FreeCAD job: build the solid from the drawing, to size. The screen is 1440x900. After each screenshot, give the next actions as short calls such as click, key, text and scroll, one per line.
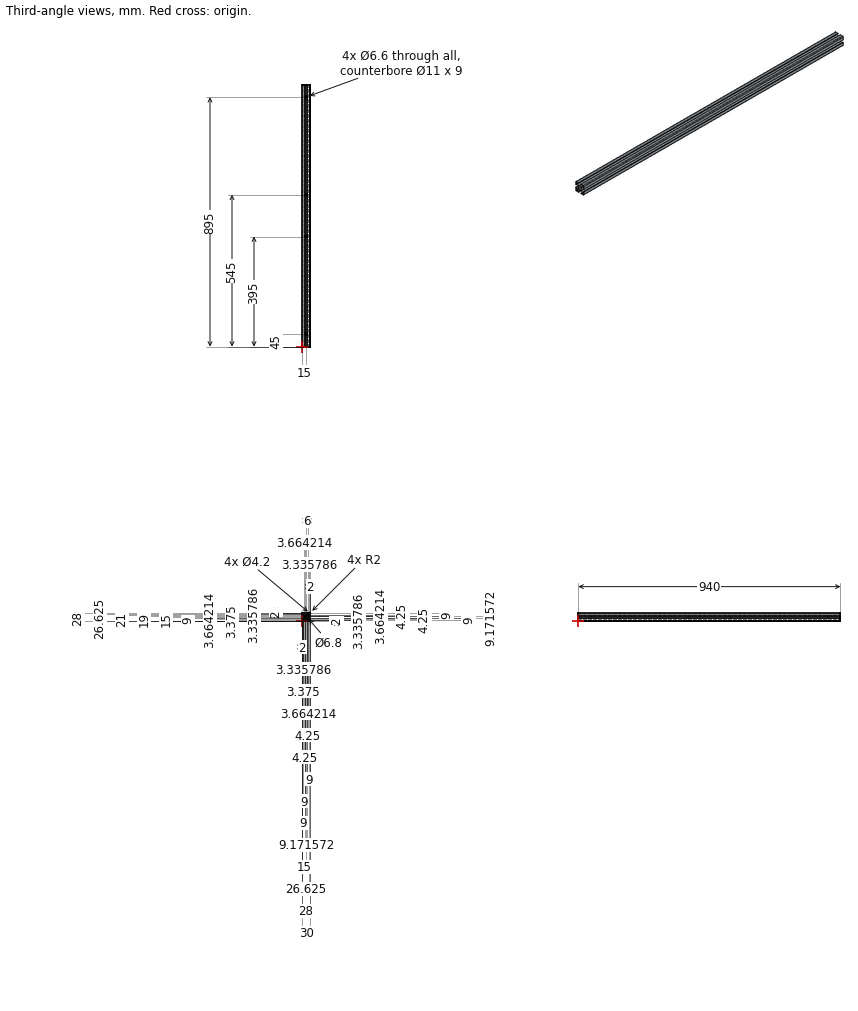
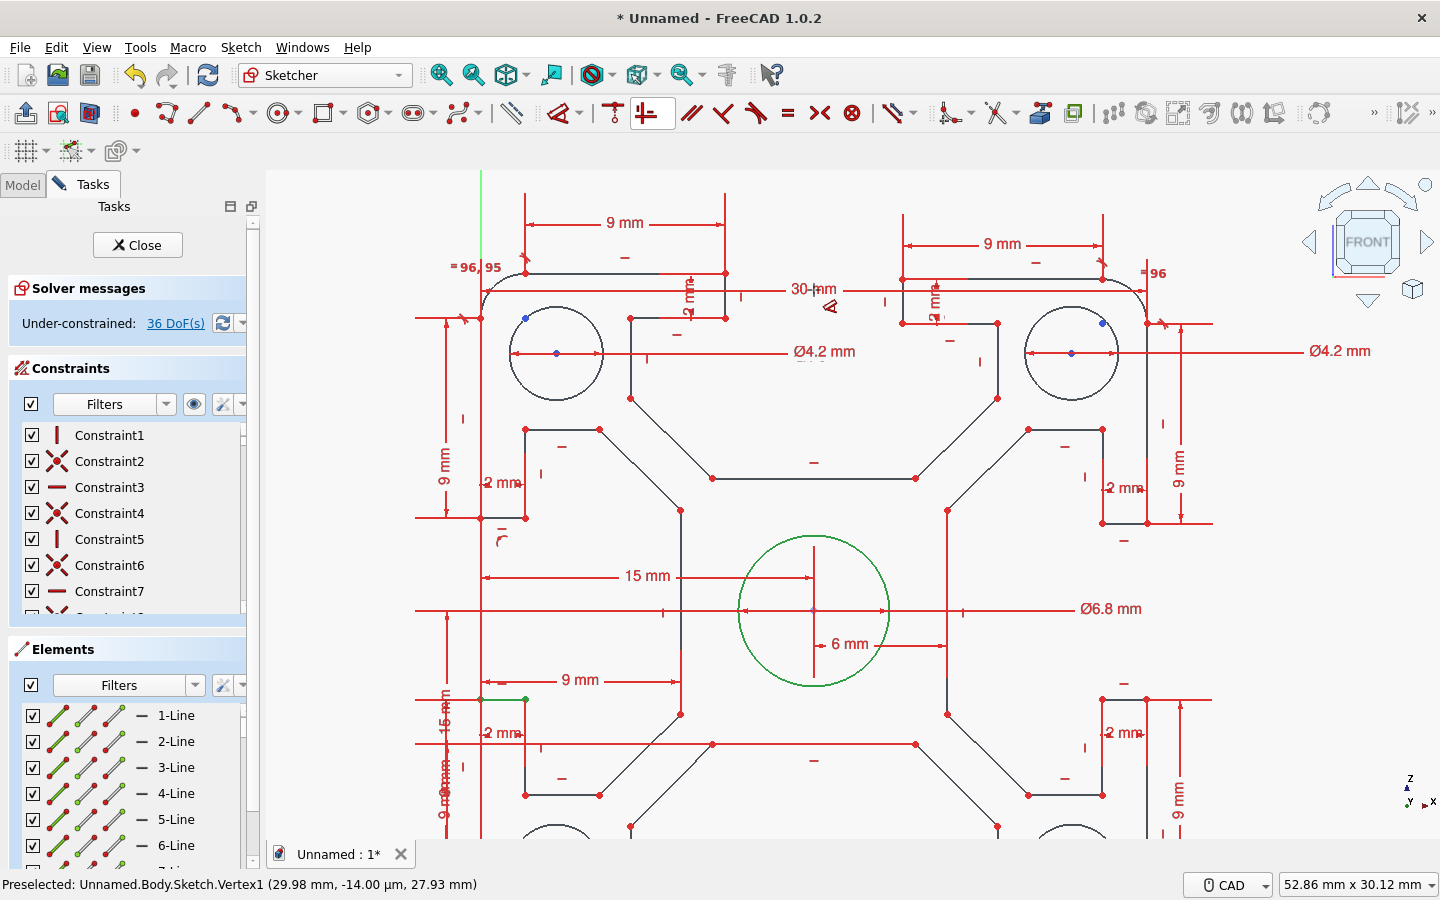
click(1147, 324)
click(1181, 567)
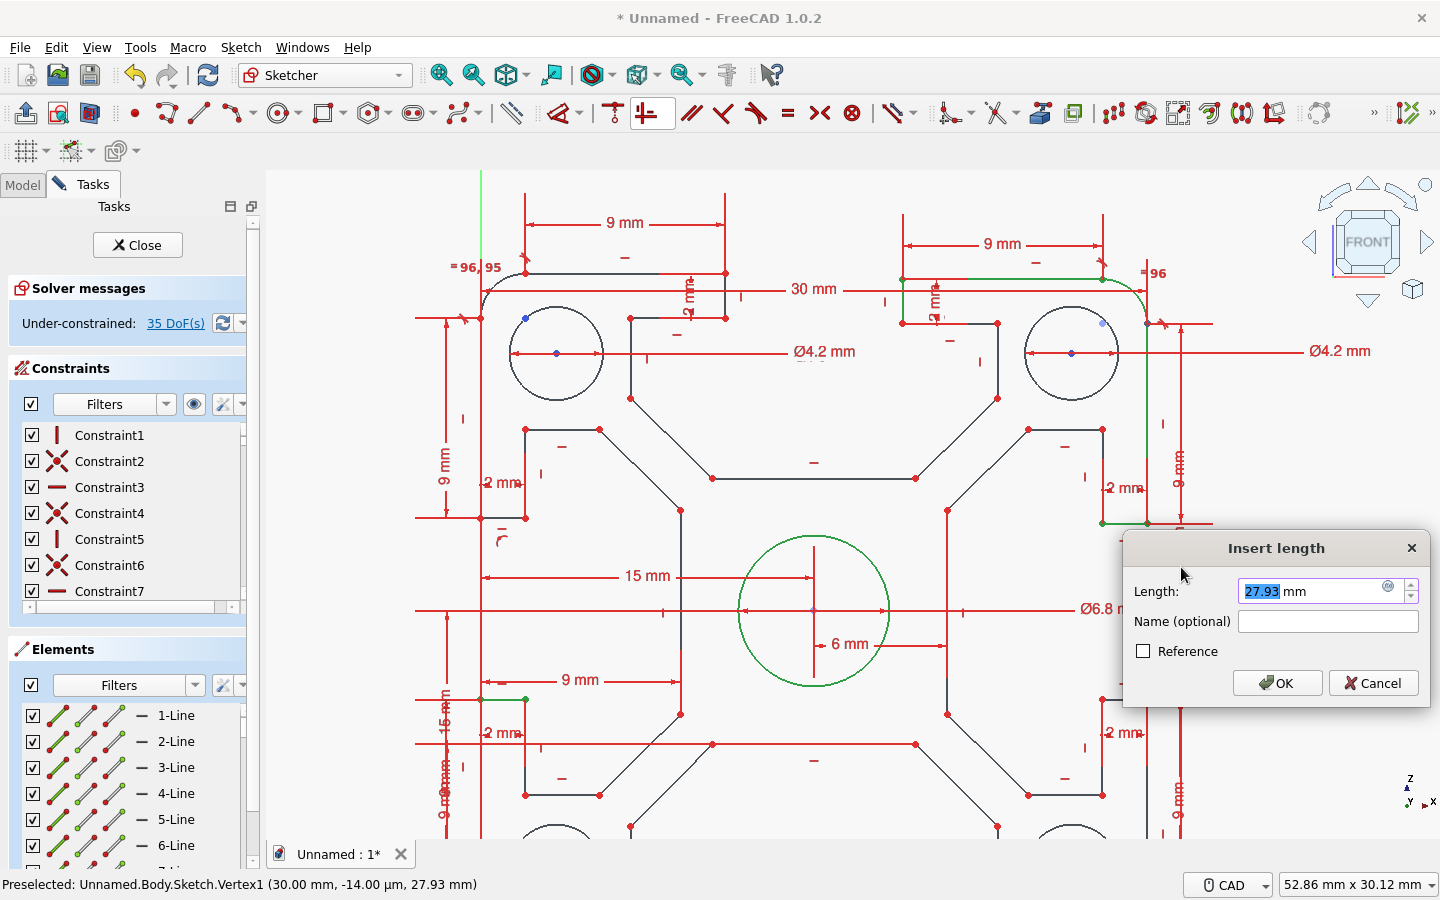
text(28)
key(Return)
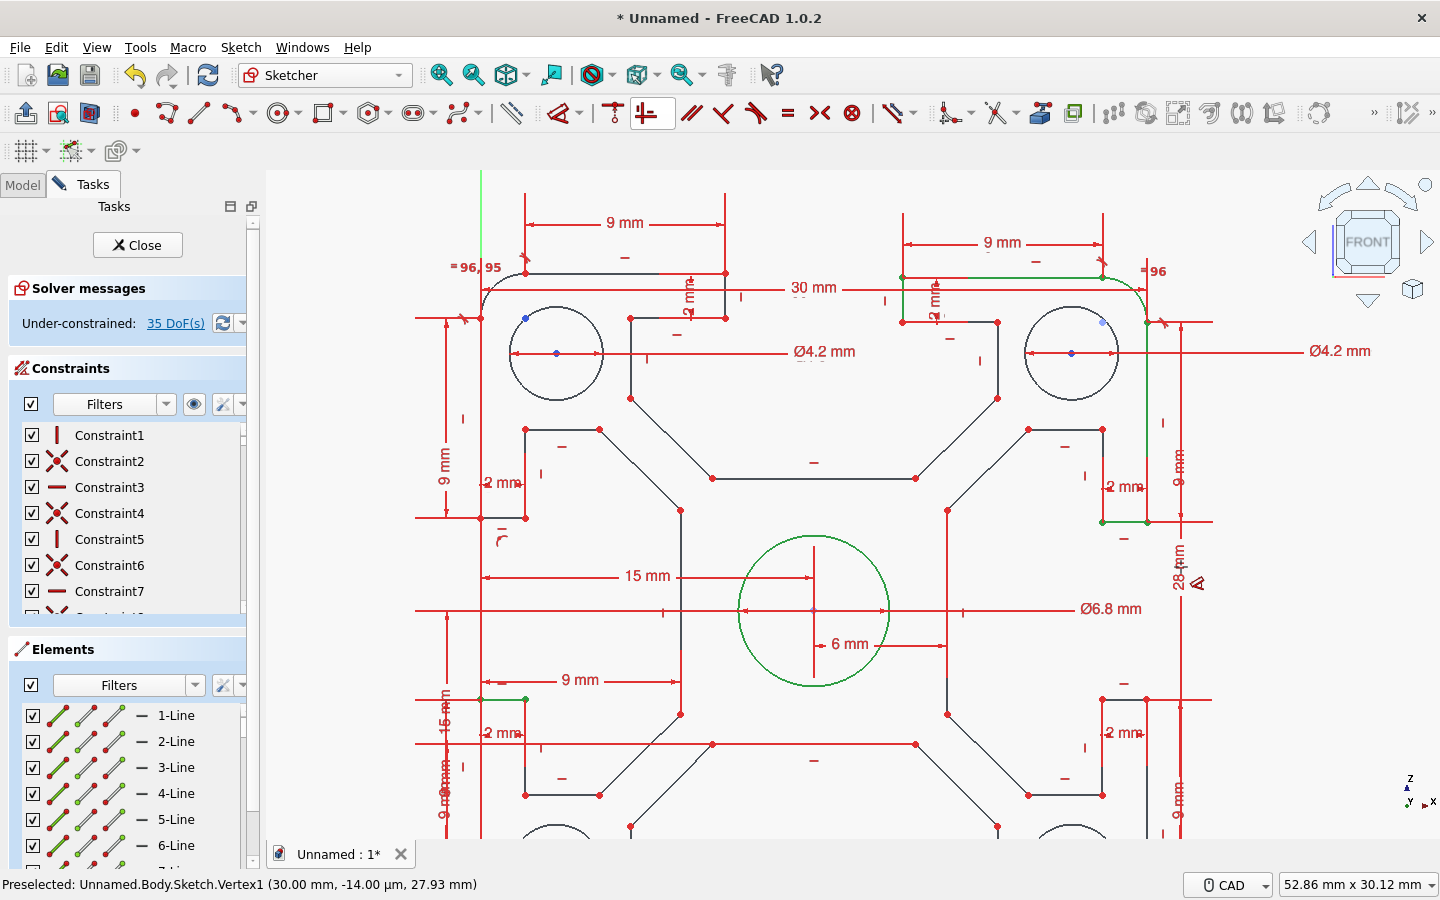
click(1102, 795)
click(791, 761)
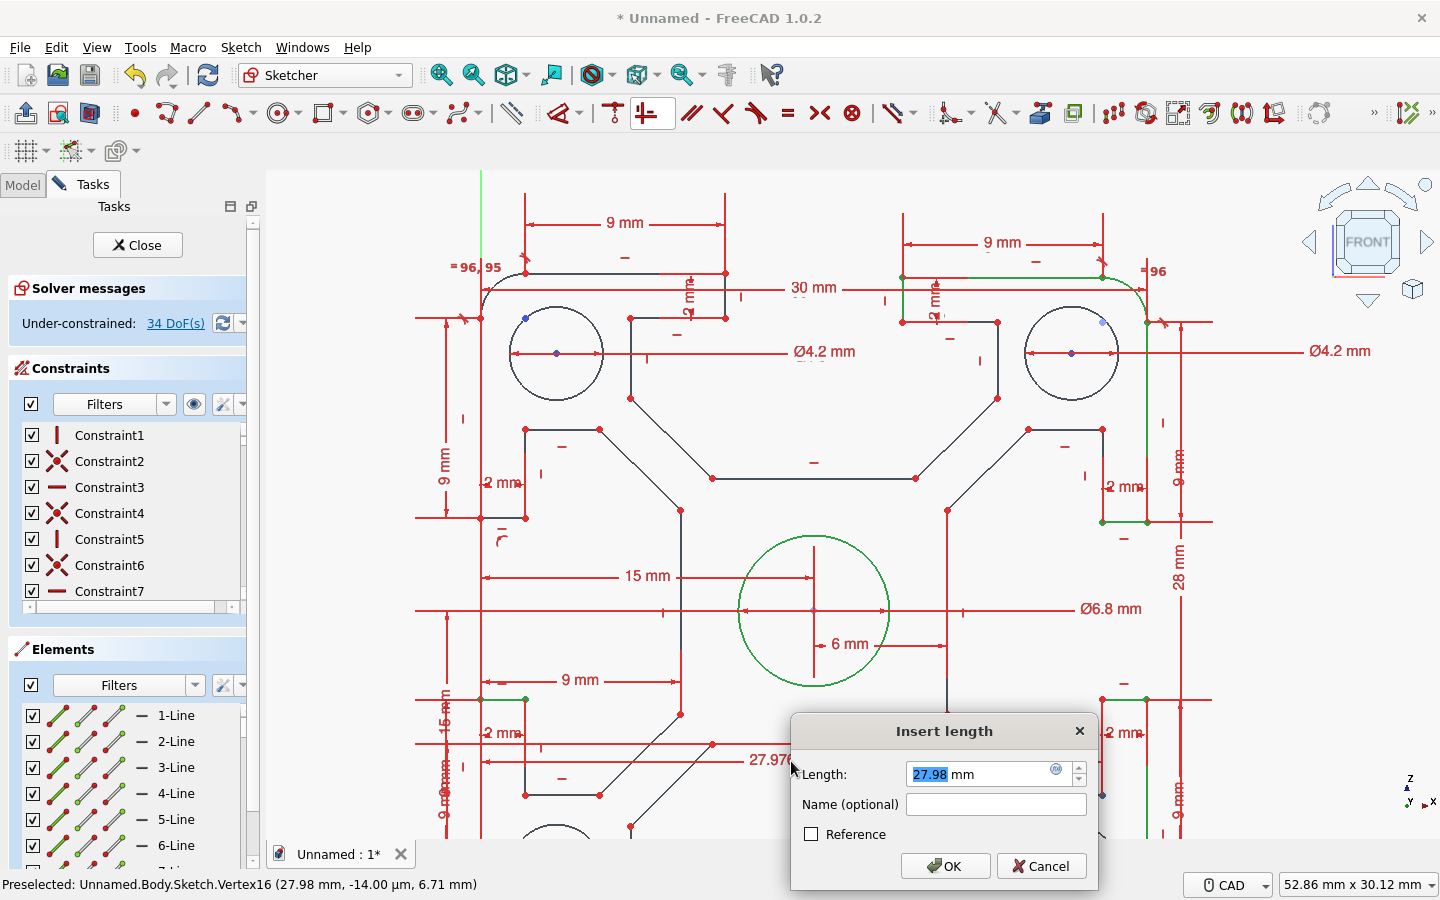
text(28)
key(Return)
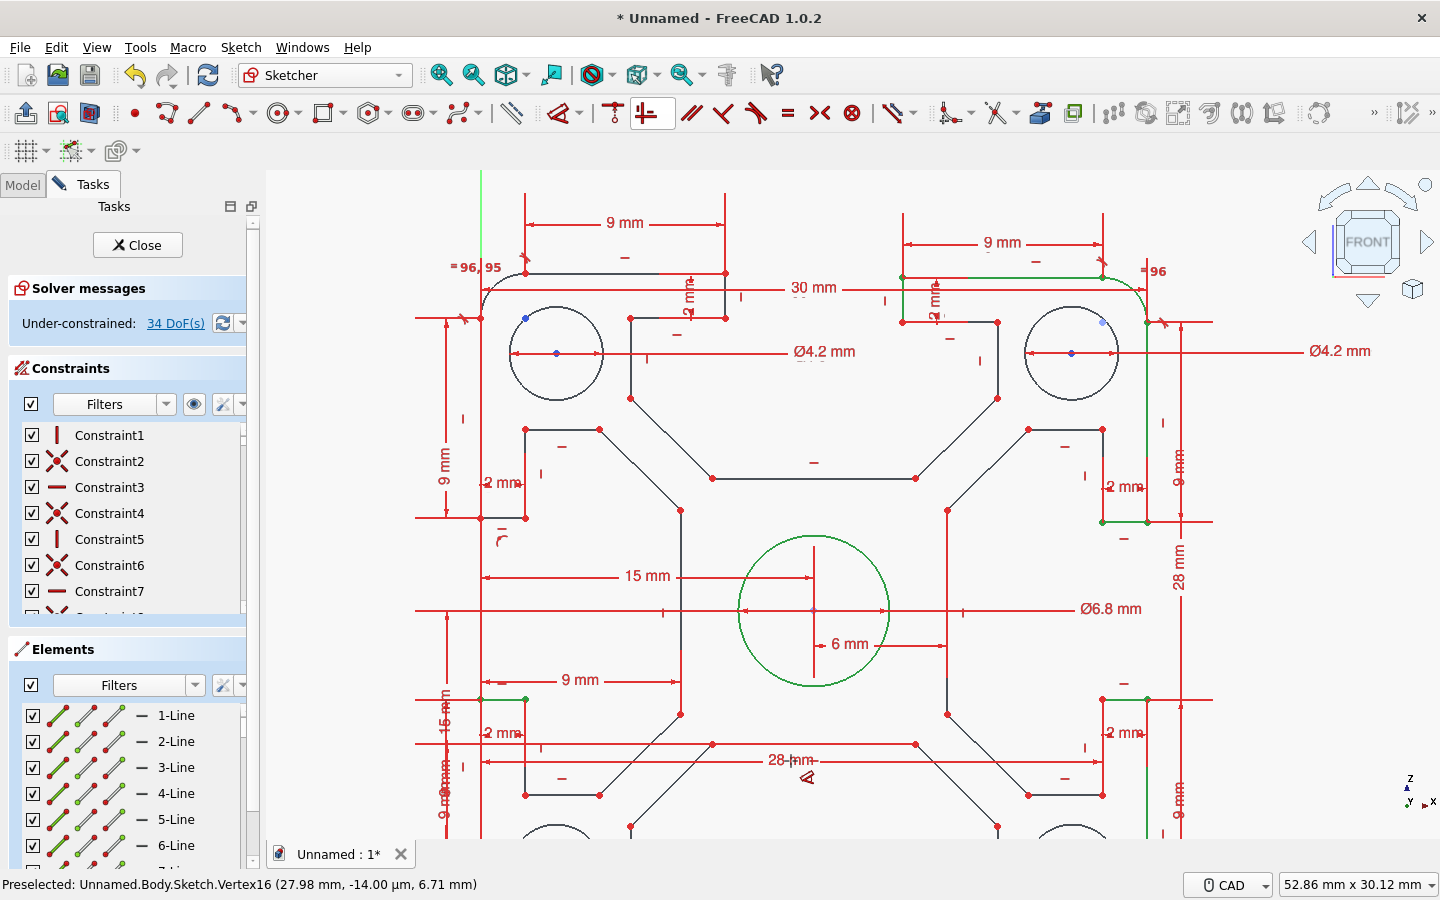
click(525, 518)
click(447, 665)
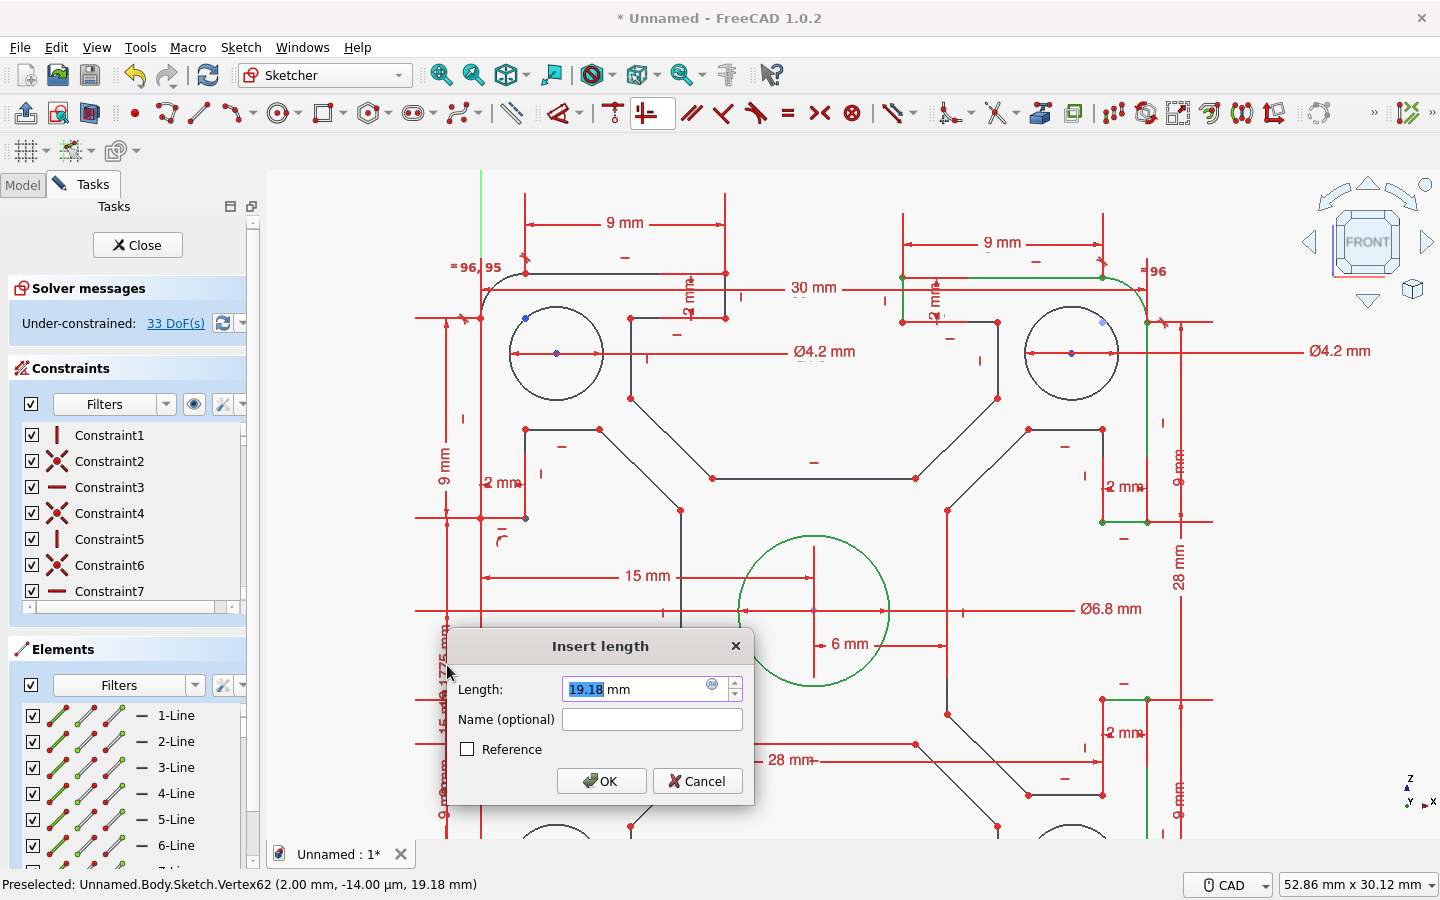
text(19)
key(Return)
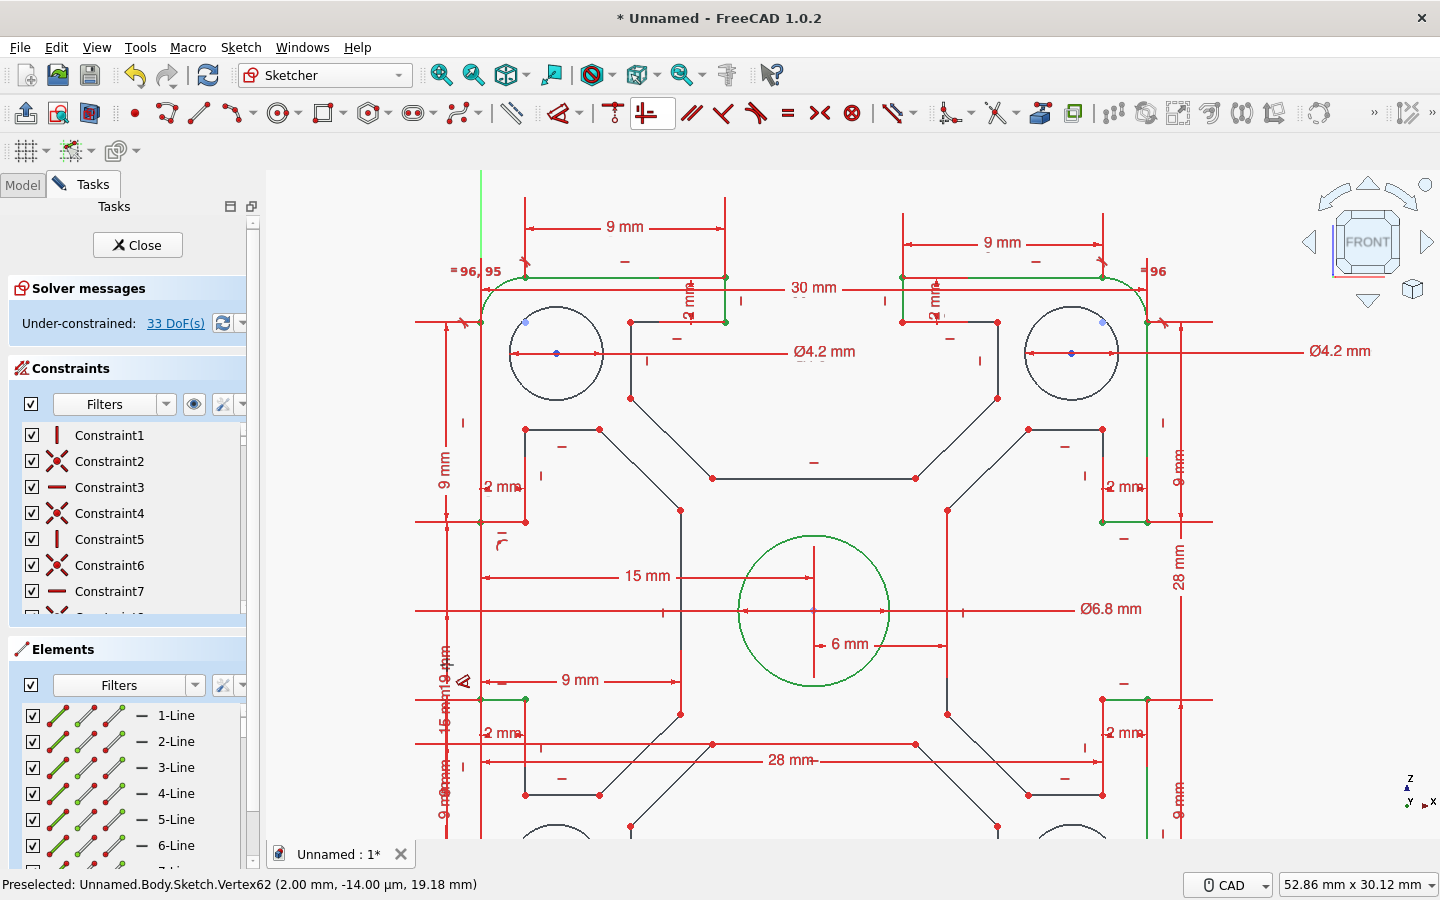
click(713, 479)
click(447, 569)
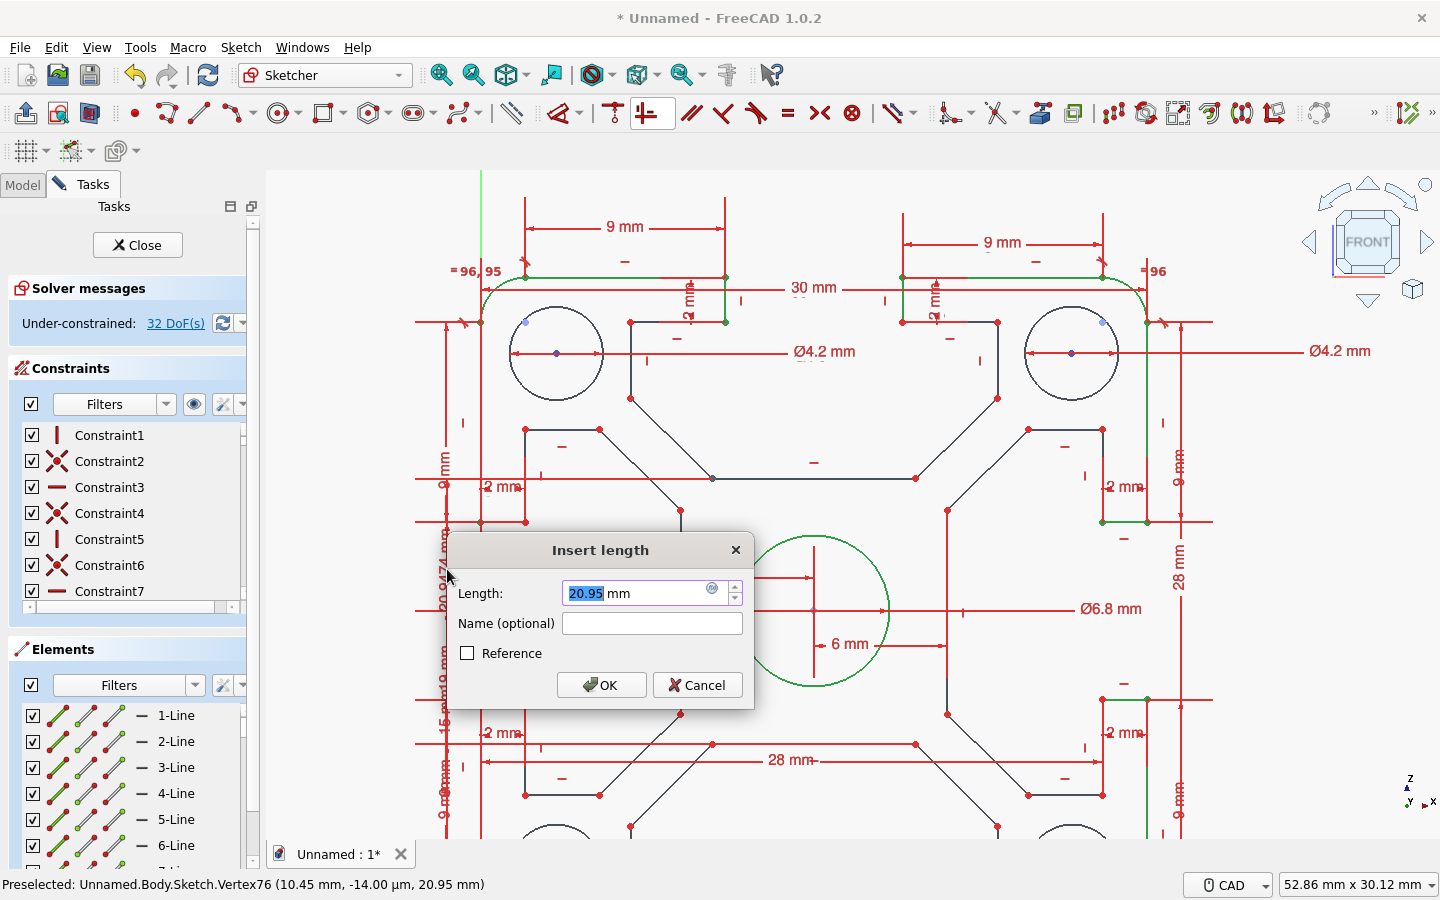
text(21)
key(Return)